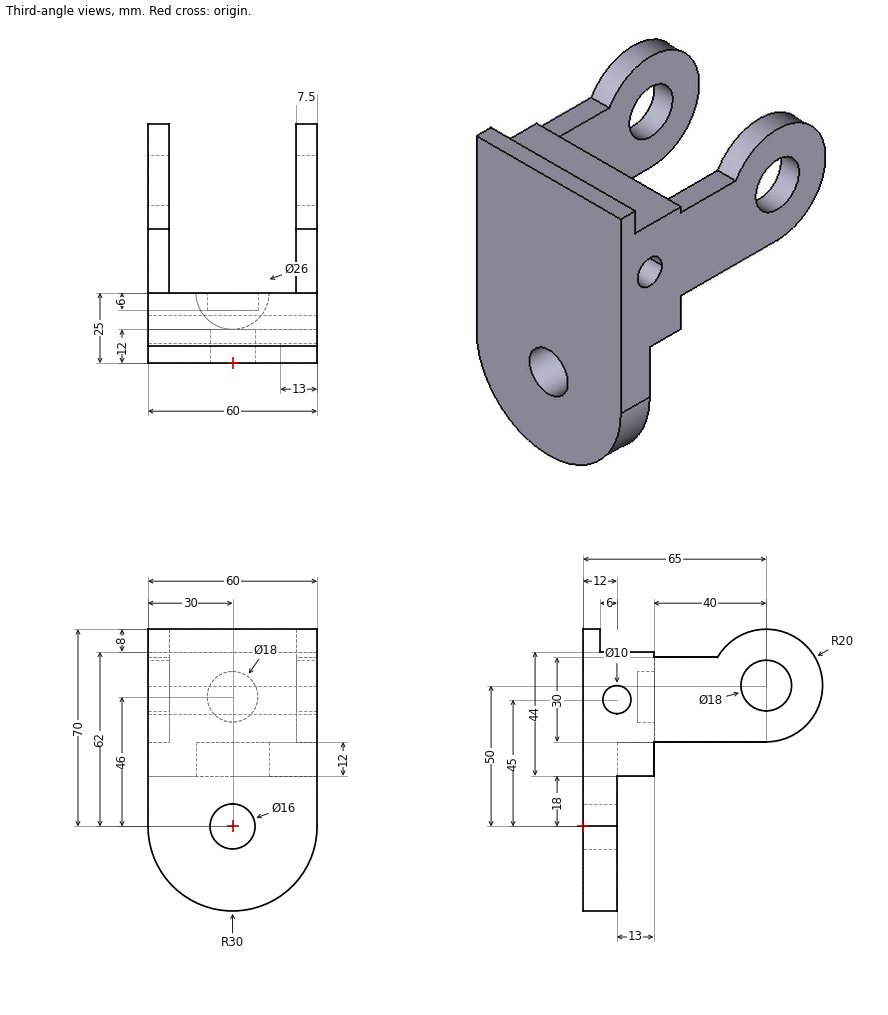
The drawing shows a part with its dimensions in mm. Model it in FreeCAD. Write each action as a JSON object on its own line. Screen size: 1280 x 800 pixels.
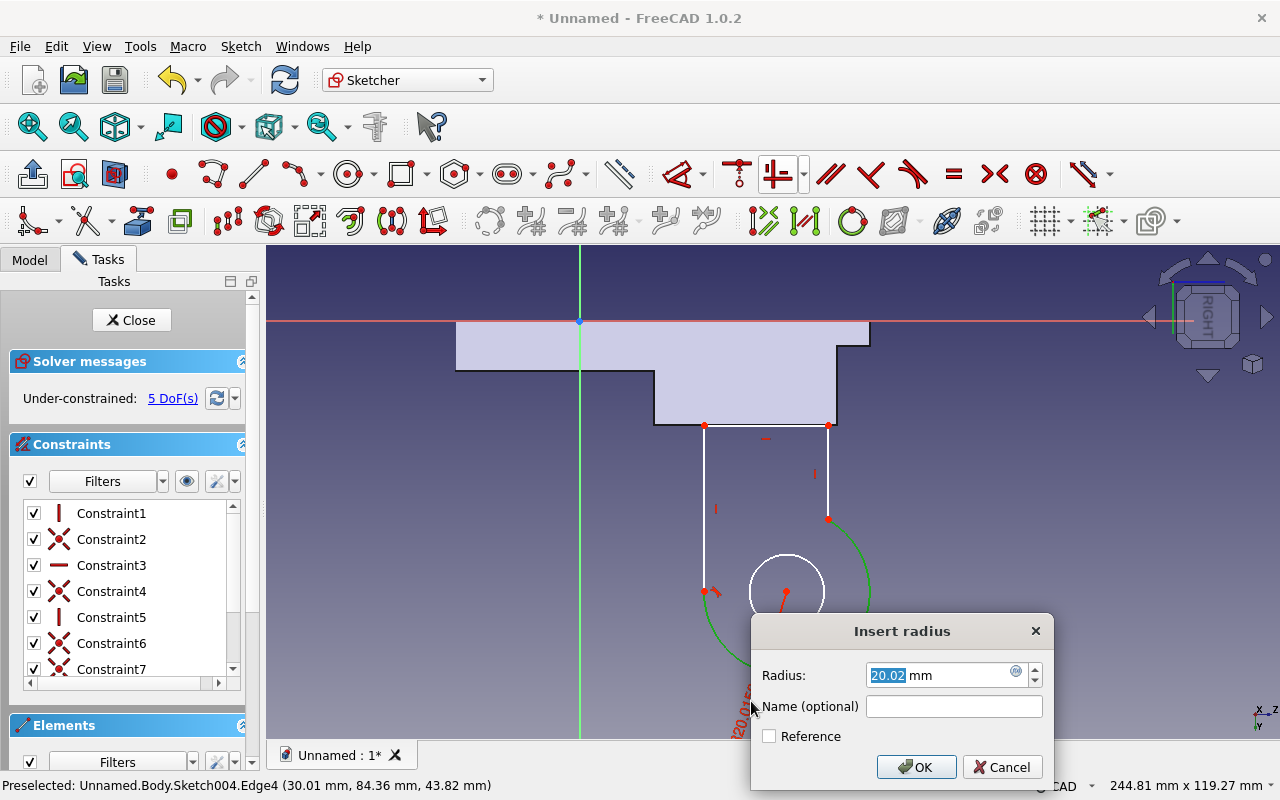
{"action": "type", "text": "20"}
{"action": "key", "text": "Return"}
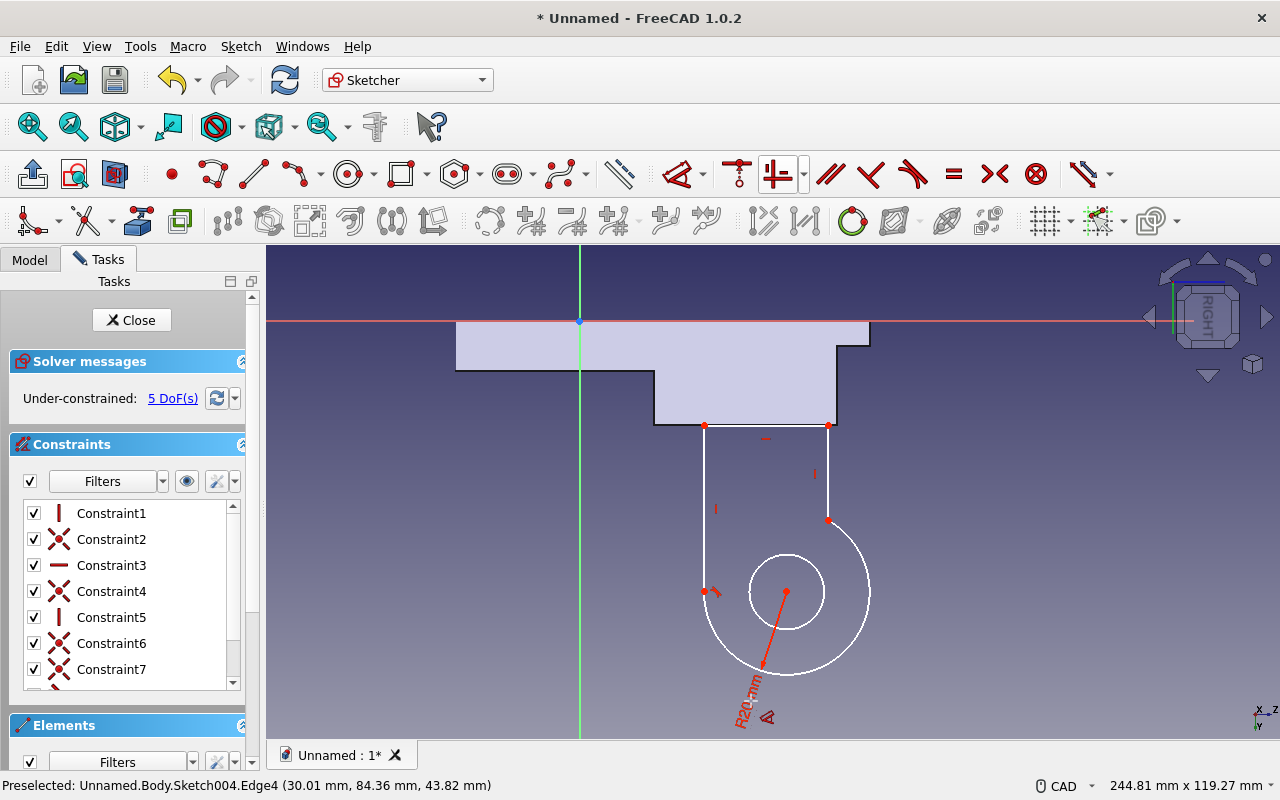
{"action": "left_click", "coordinate": [813, 565]}
{"action": "left_click", "coordinate": [835, 542]}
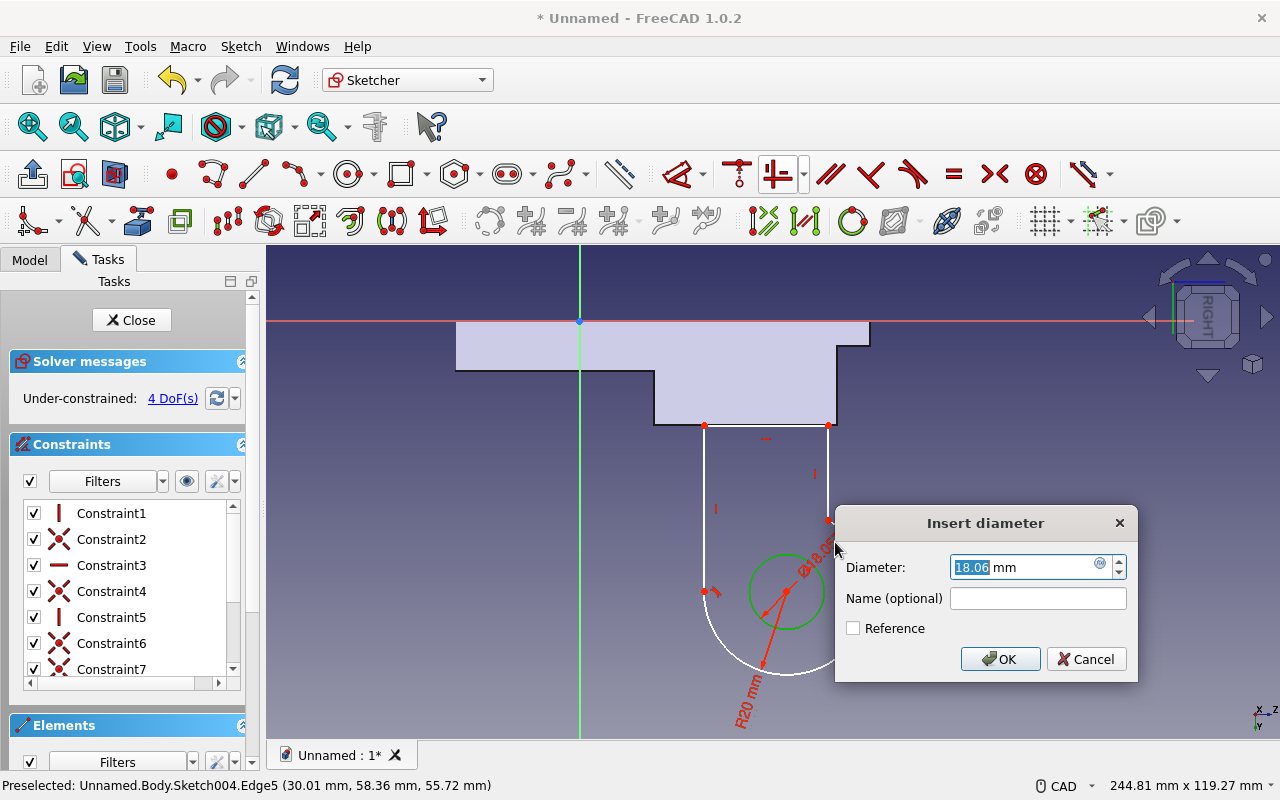
{"action": "type", "text": "18"}
{"action": "key", "text": "Return"}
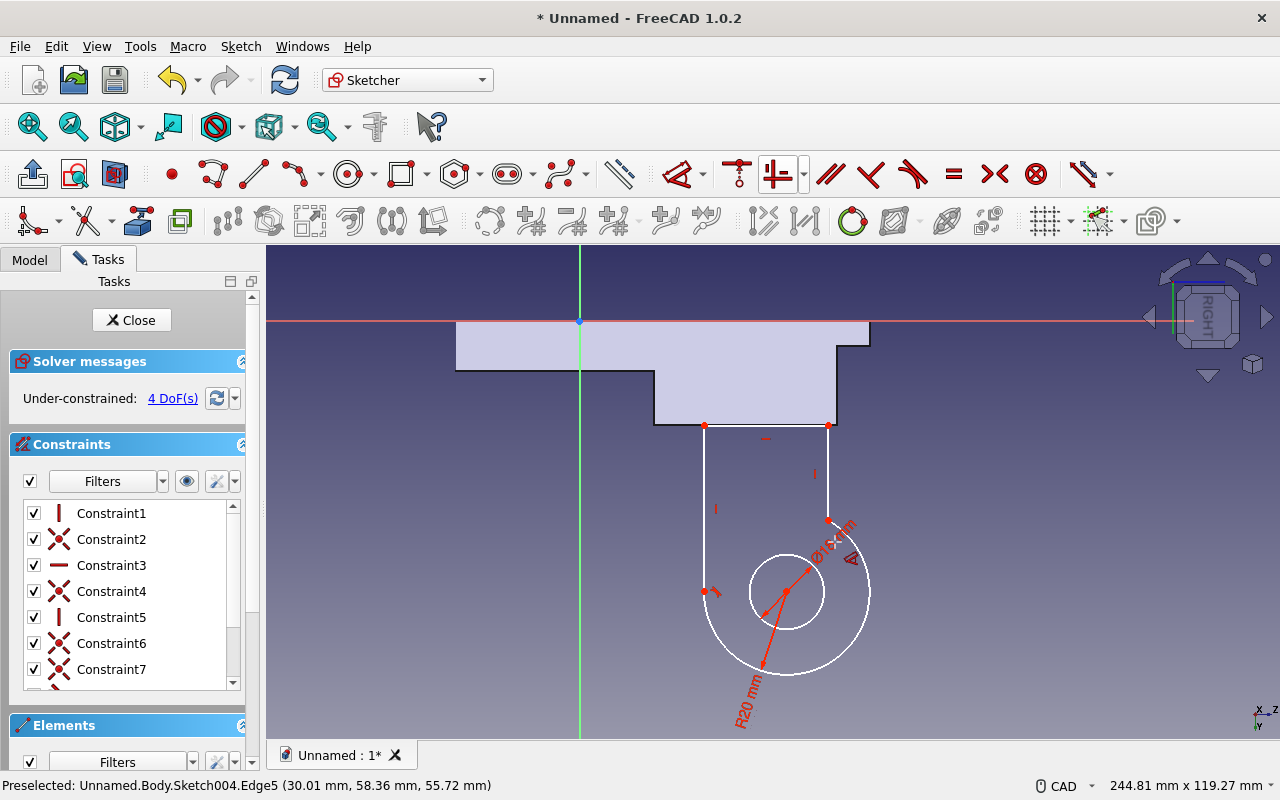
{"action": "left_click", "coordinate": [791, 426]}
{"action": "left_click", "coordinate": [766, 392]}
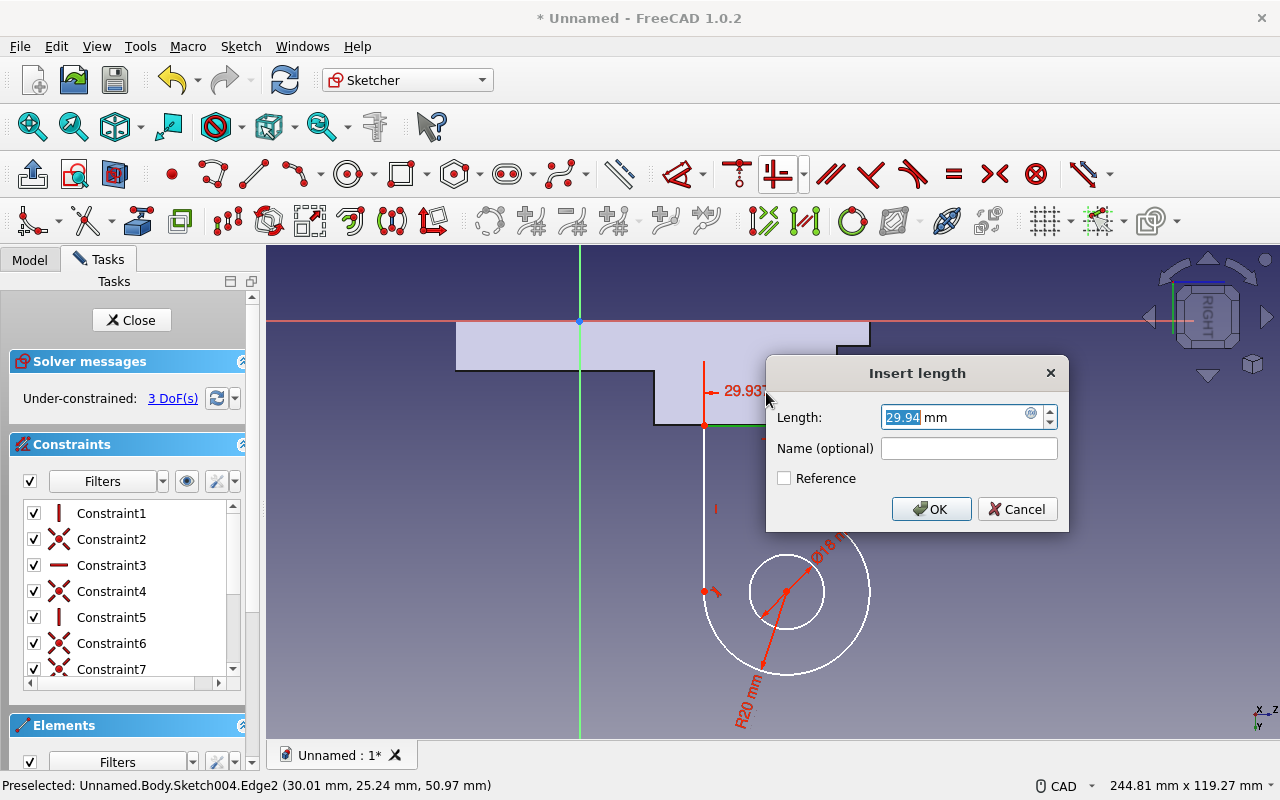
{"action": "type", "text": "30"}
{"action": "key", "text": "Return"}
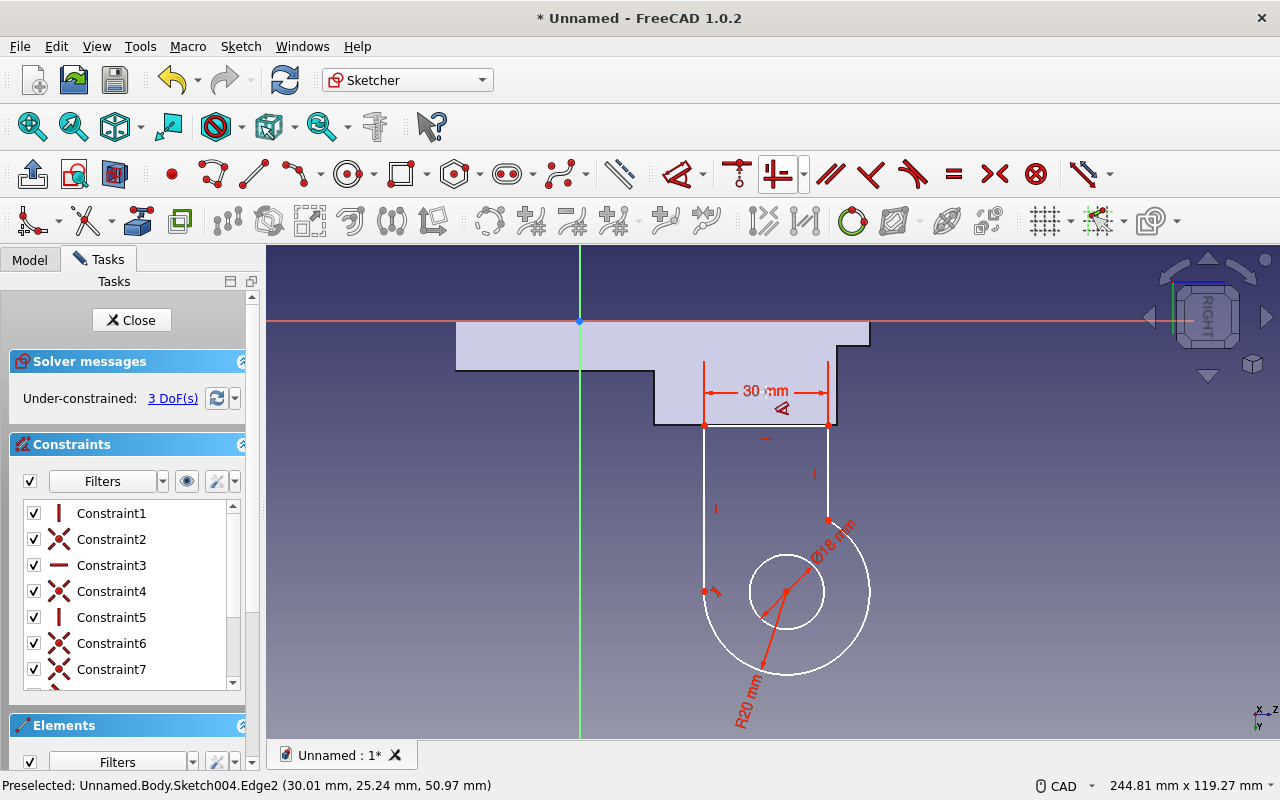
{"action": "left_click", "coordinate": [704, 476]}
{"action": "left_click", "coordinate": [670, 509]}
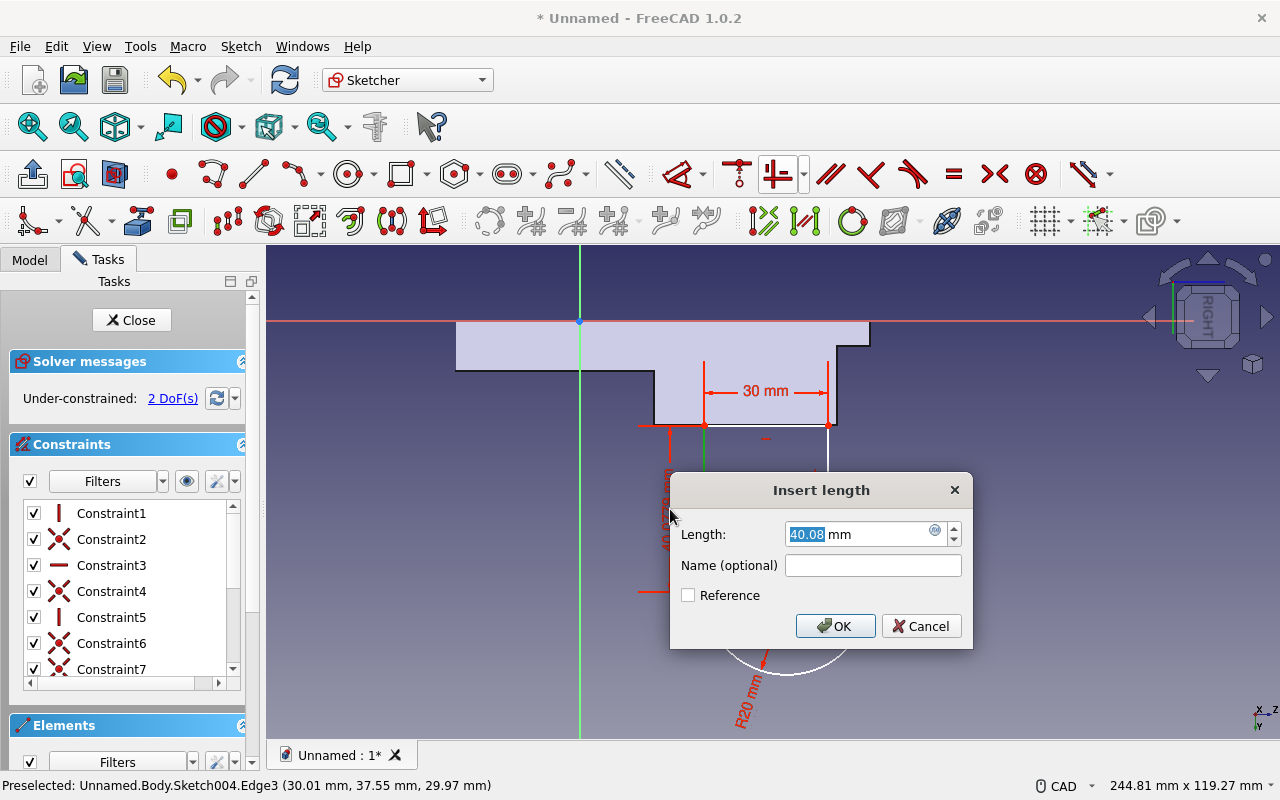
{"action": "type", "text": "40"}
{"action": "key", "text": "Return"}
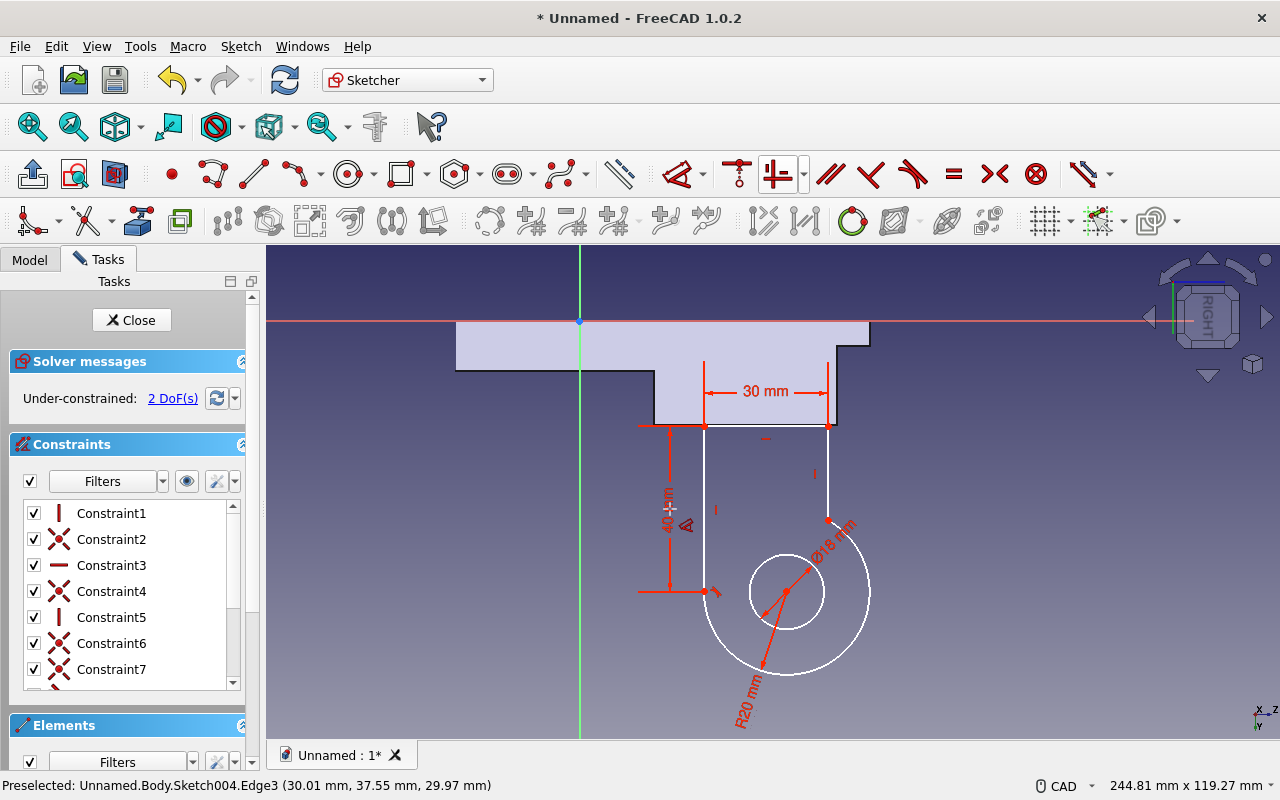
{"action": "left_click", "coordinate": [787, 592]}
{"action": "left_click", "coordinate": [683, 287]}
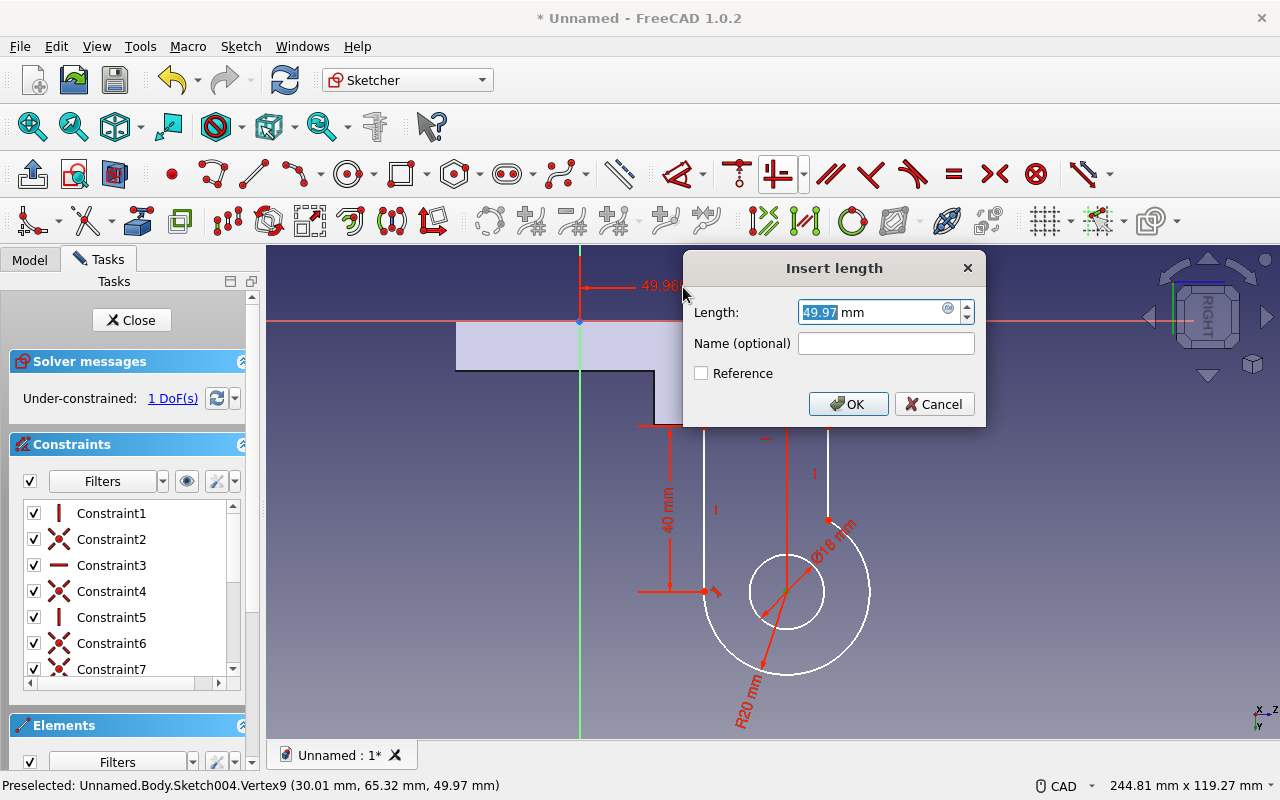
{"action": "type", "text": "50"}
{"action": "key", "text": "Return"}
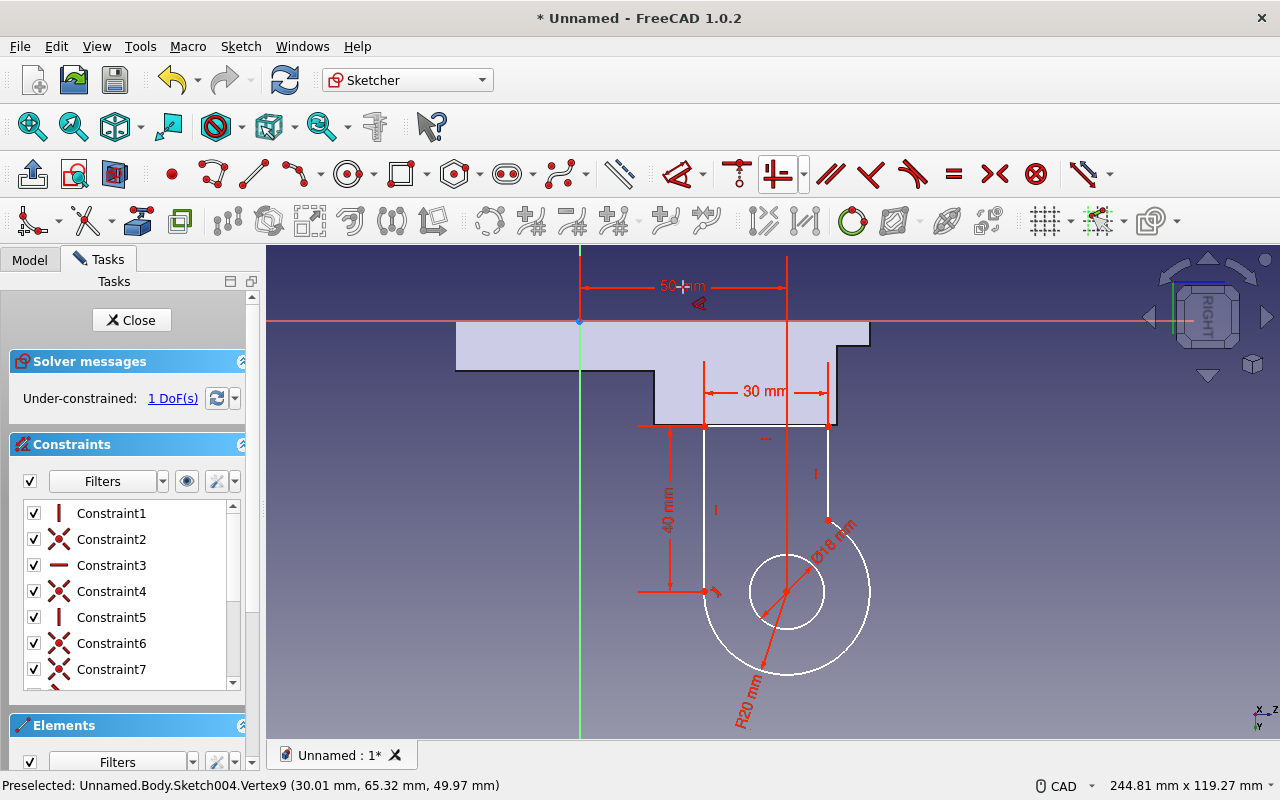
{"action": "left_click", "coordinate": [787, 592]}
{"action": "left_click", "coordinate": [546, 457]}